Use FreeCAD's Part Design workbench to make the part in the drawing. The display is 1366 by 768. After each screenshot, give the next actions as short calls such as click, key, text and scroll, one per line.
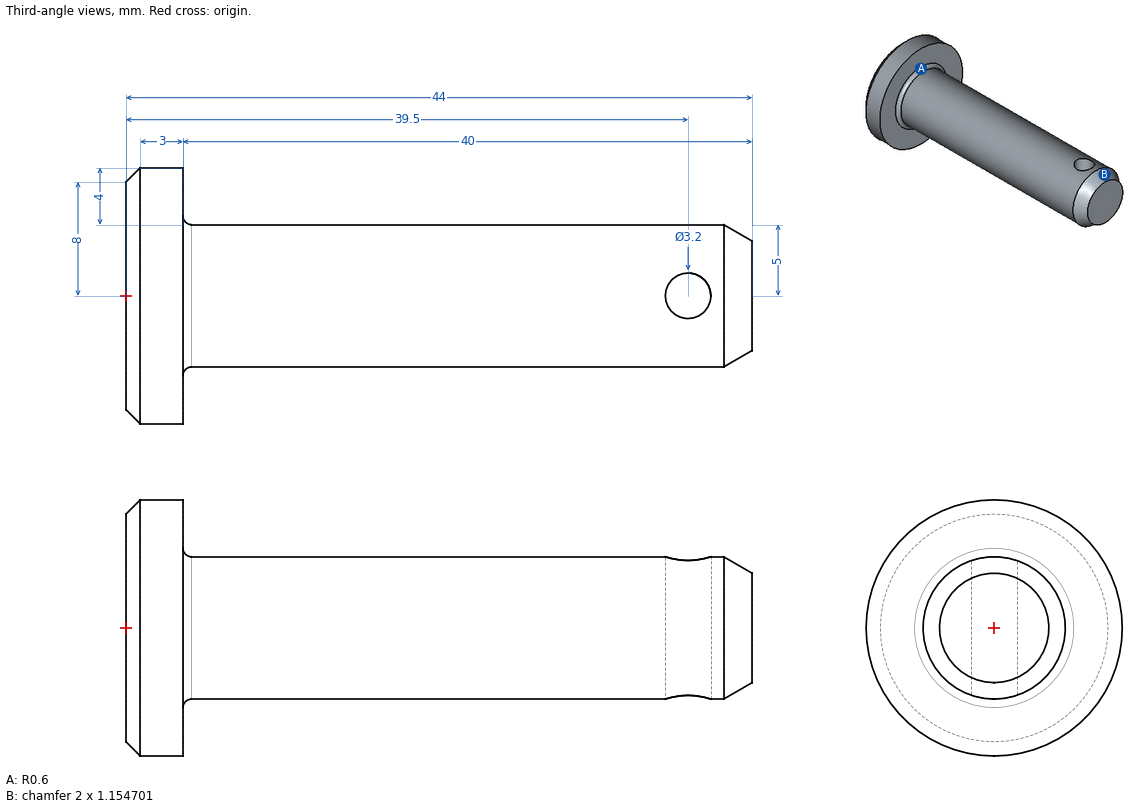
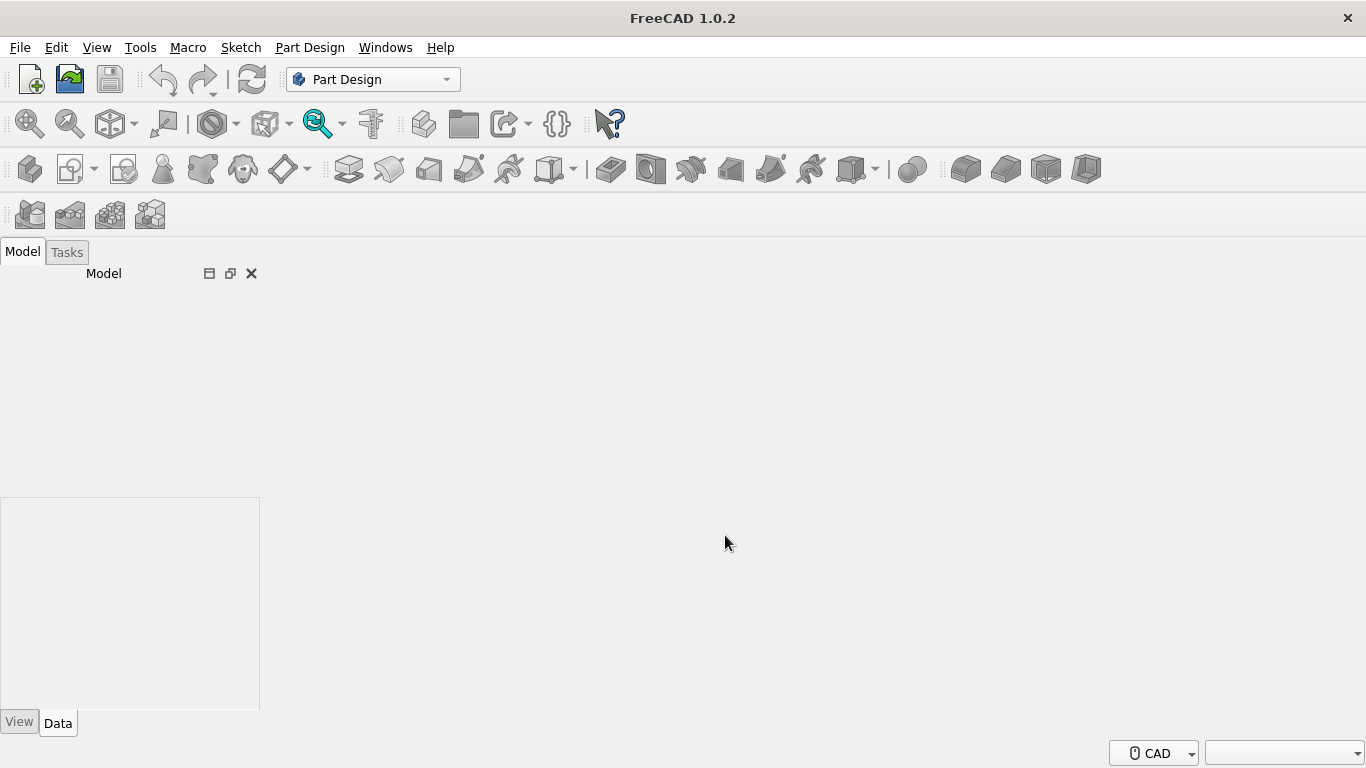
key(ctrl+n)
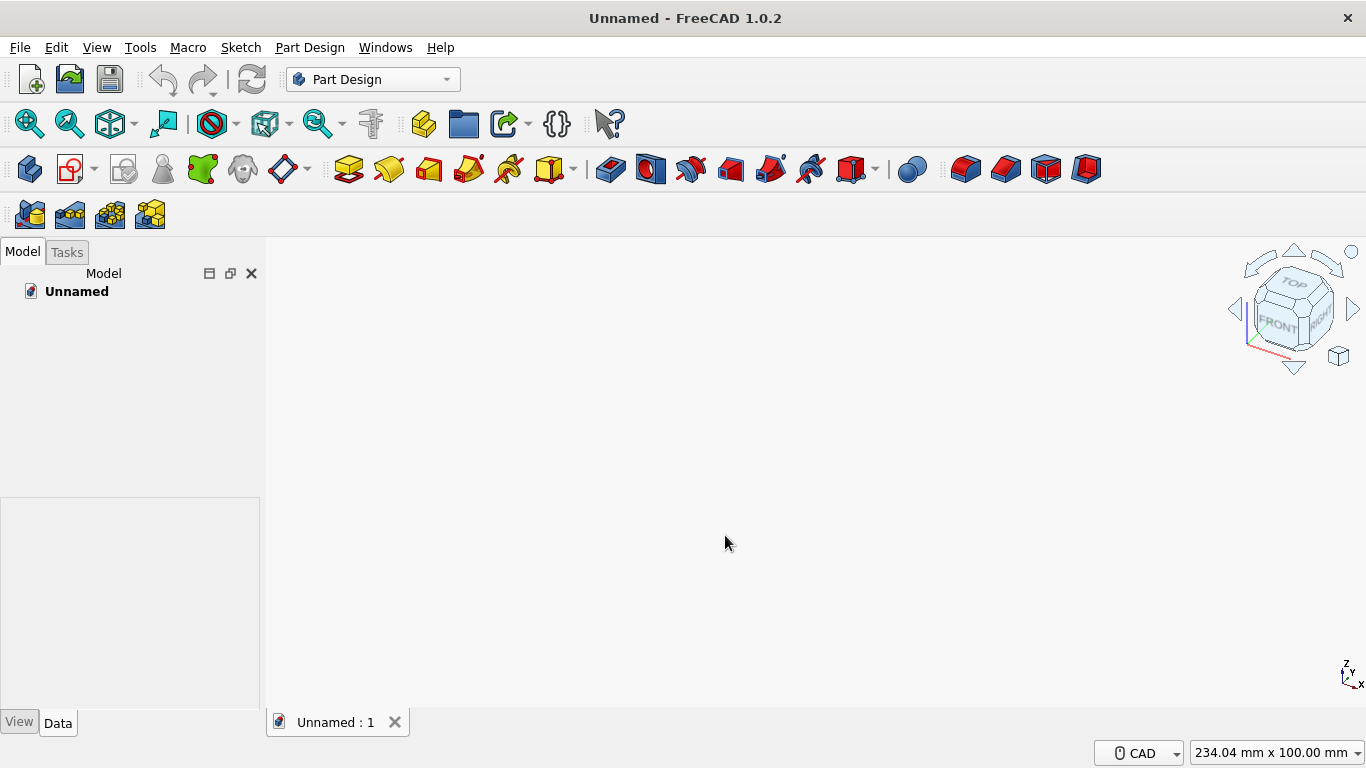
click(70, 170)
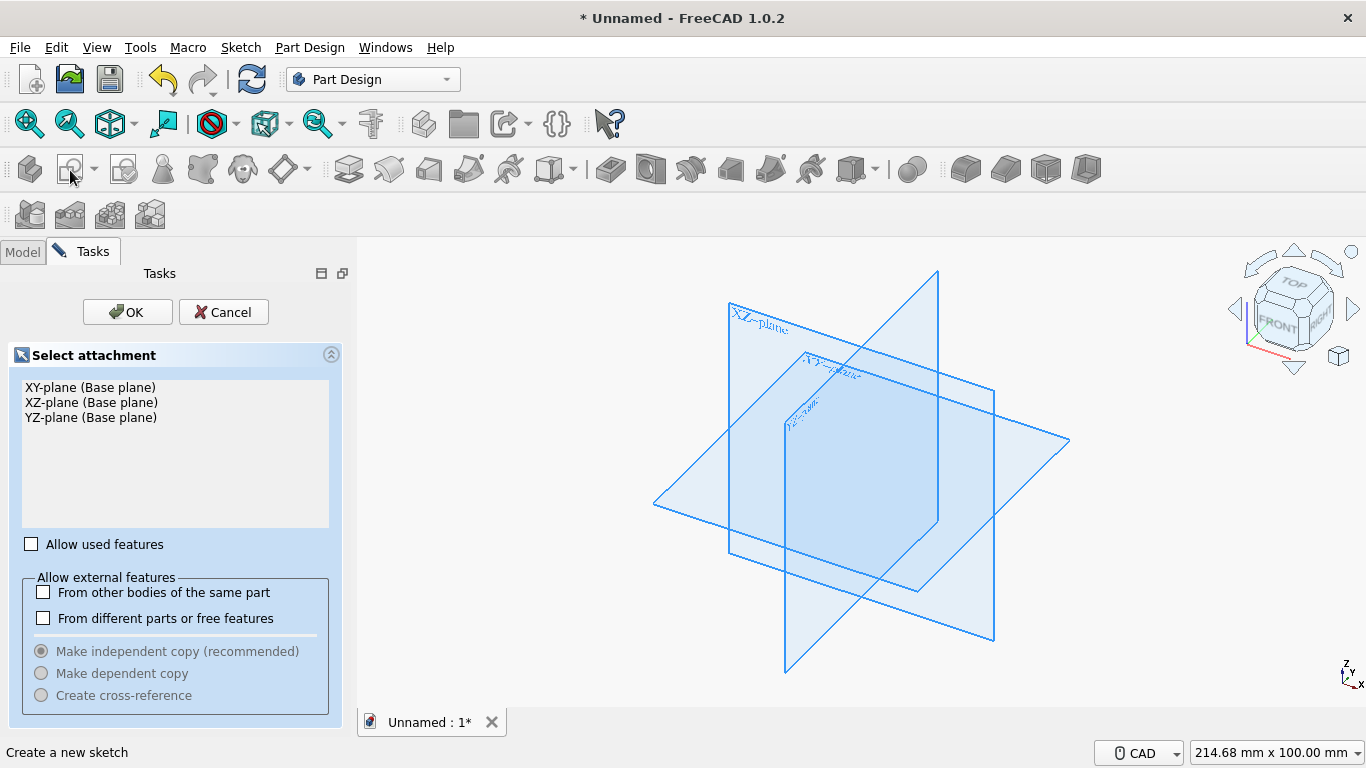
click(82, 388)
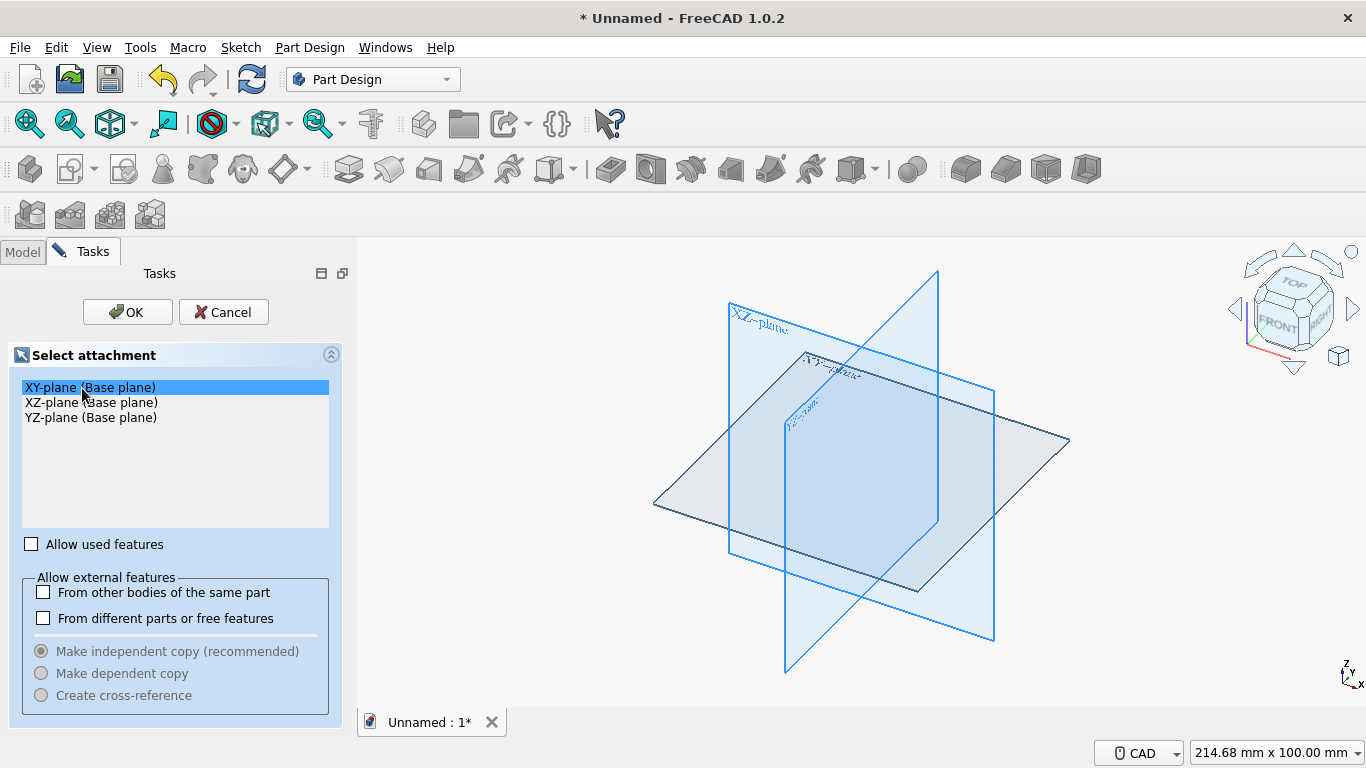
click(128, 312)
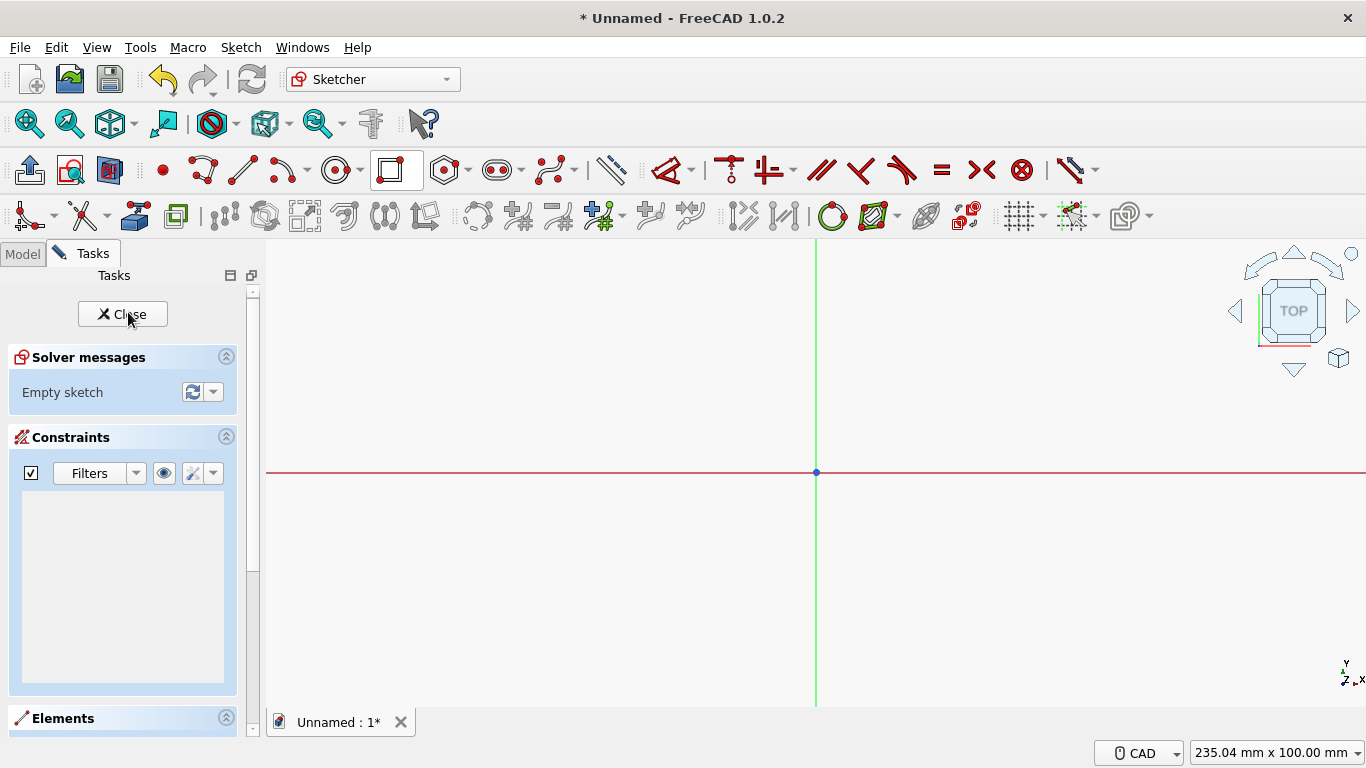
scroll(993, 443, up, 6)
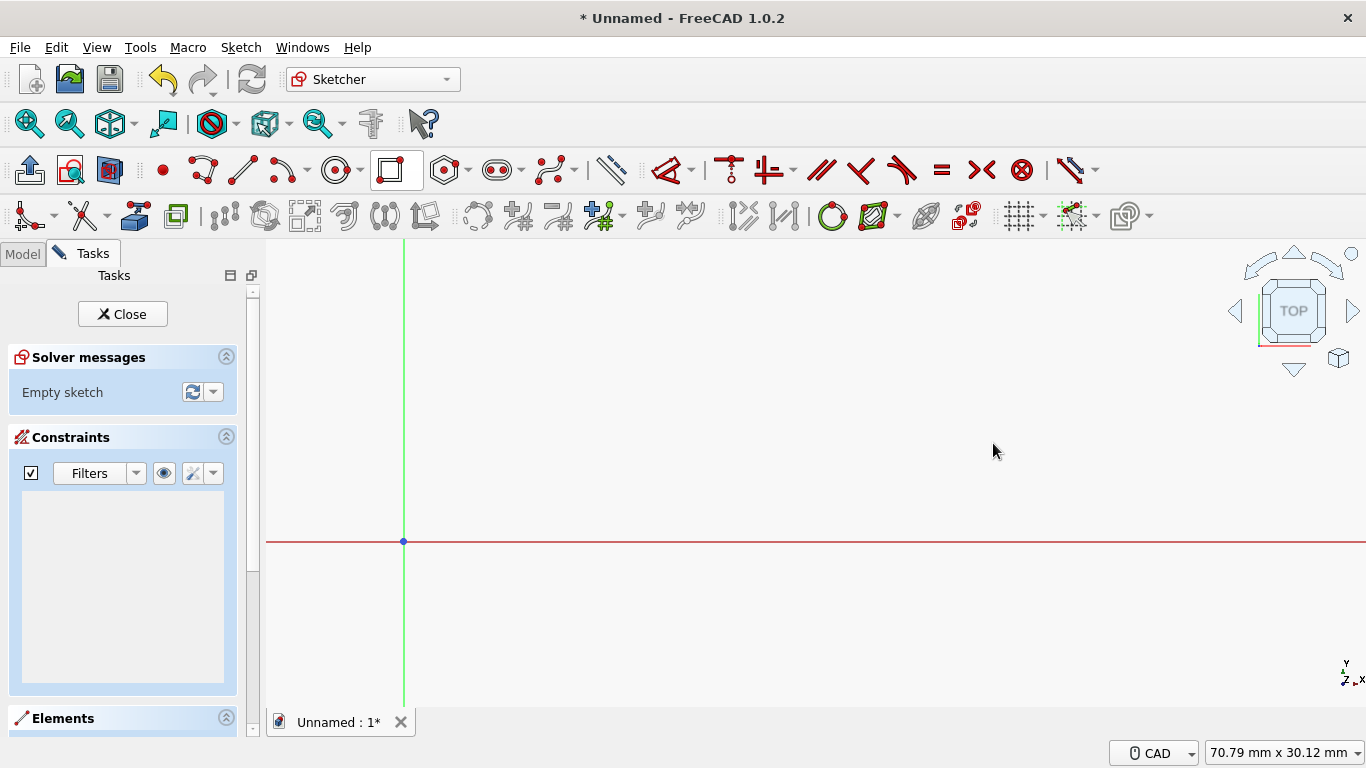
key(g)
key(m)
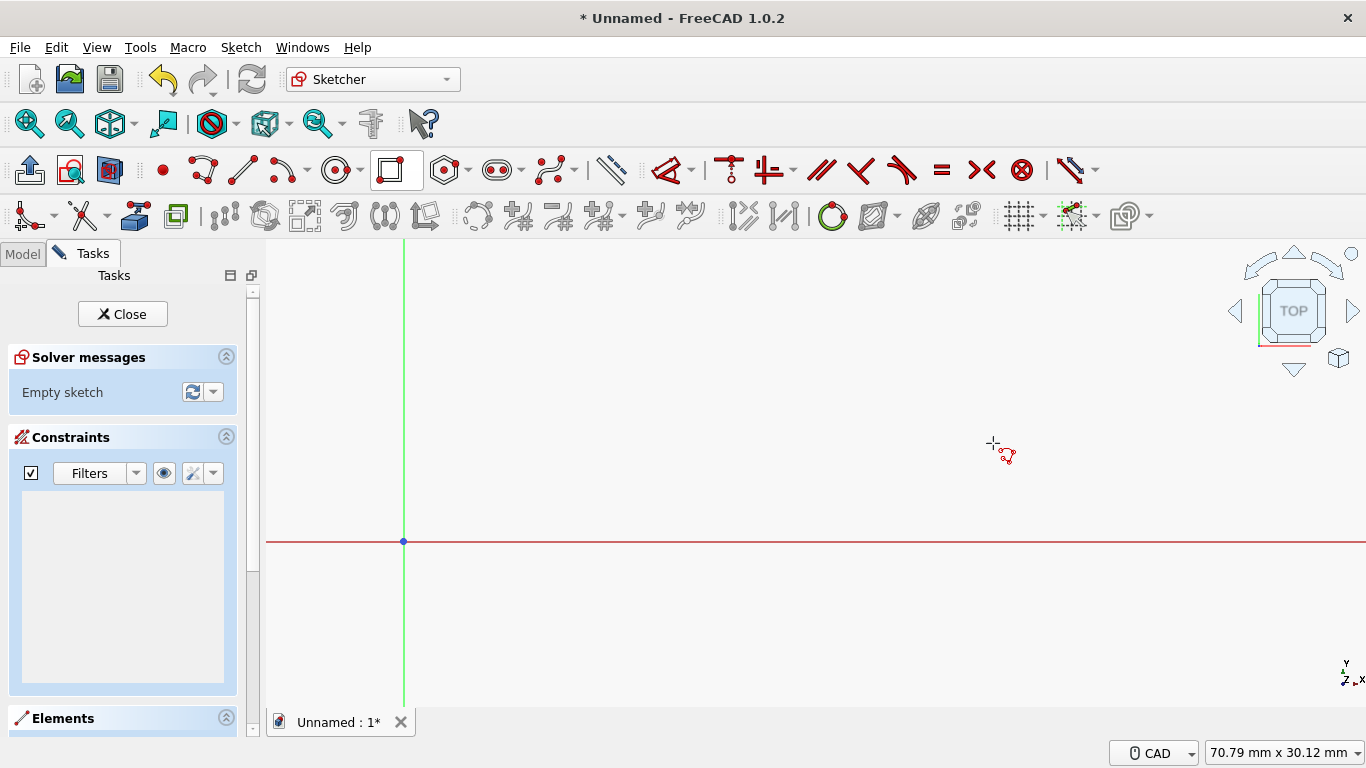
click(404, 542)
click(1087, 533)
click(1087, 464)
click(466, 464)
click(466, 402)
click(419, 402)
click(413, 417)
click(404, 542)
key(Escape)
key(Escape)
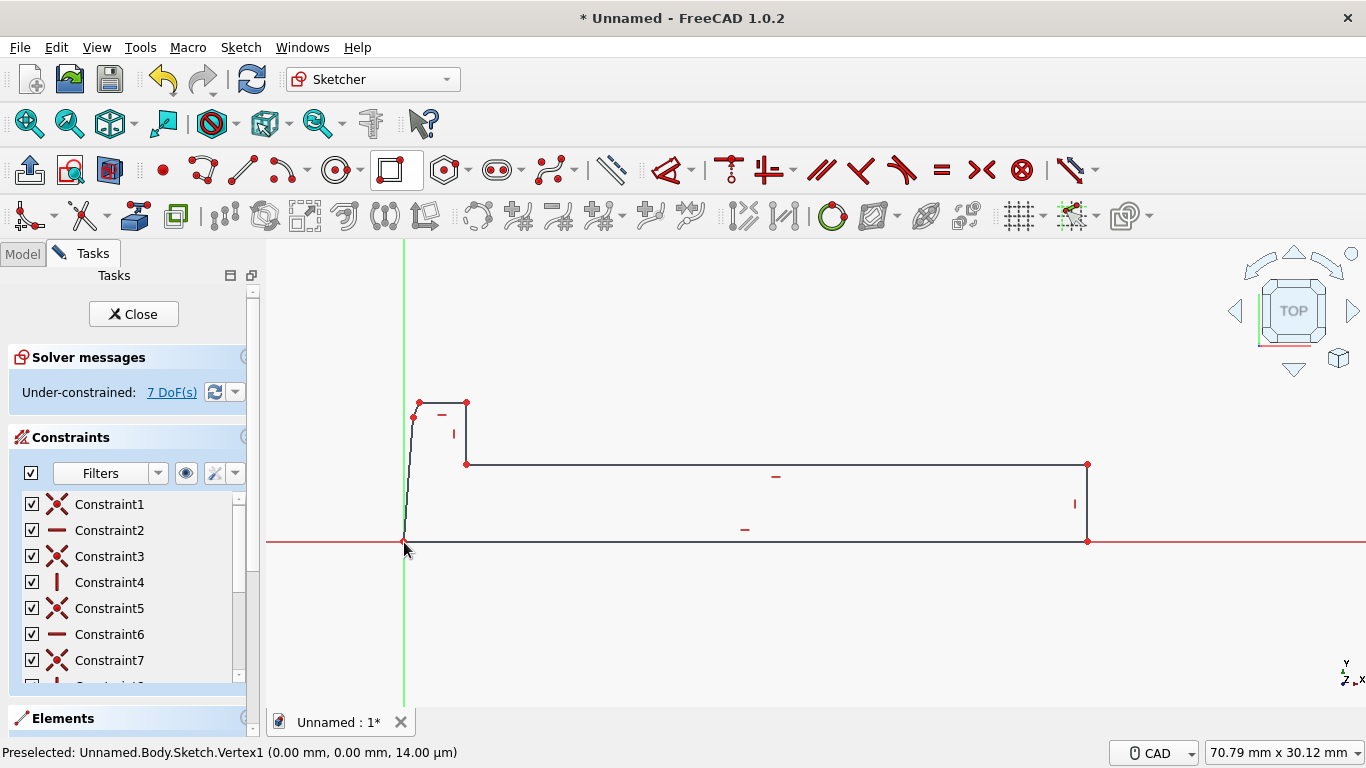
click(407, 505)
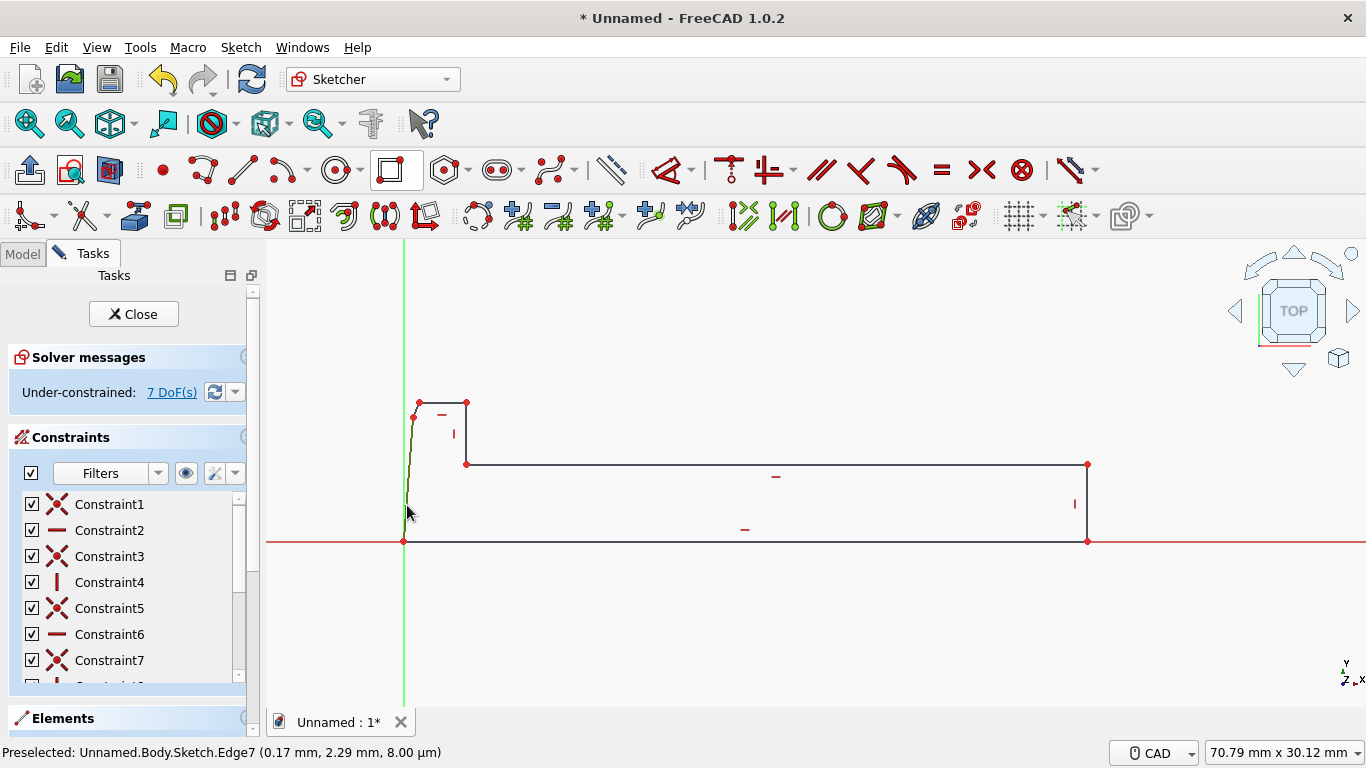
click(796, 170)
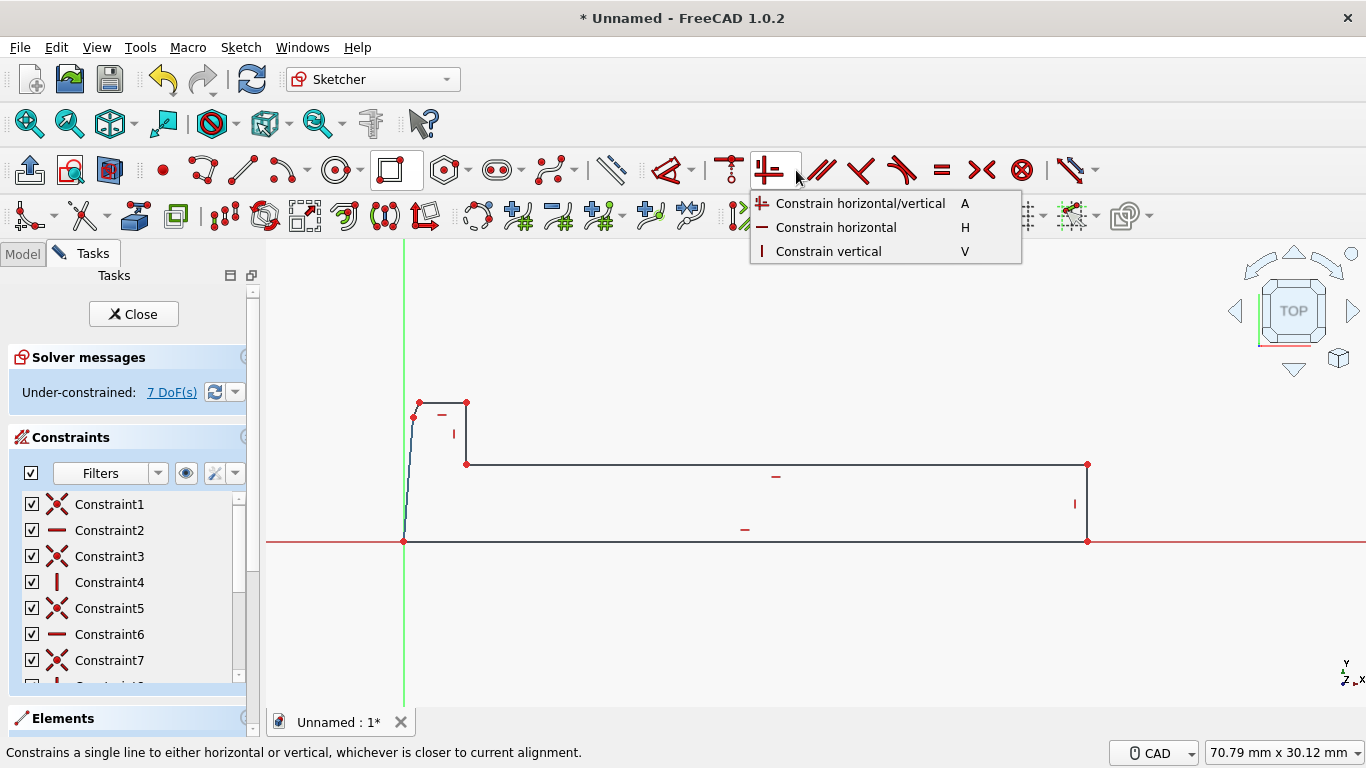
click(886, 251)